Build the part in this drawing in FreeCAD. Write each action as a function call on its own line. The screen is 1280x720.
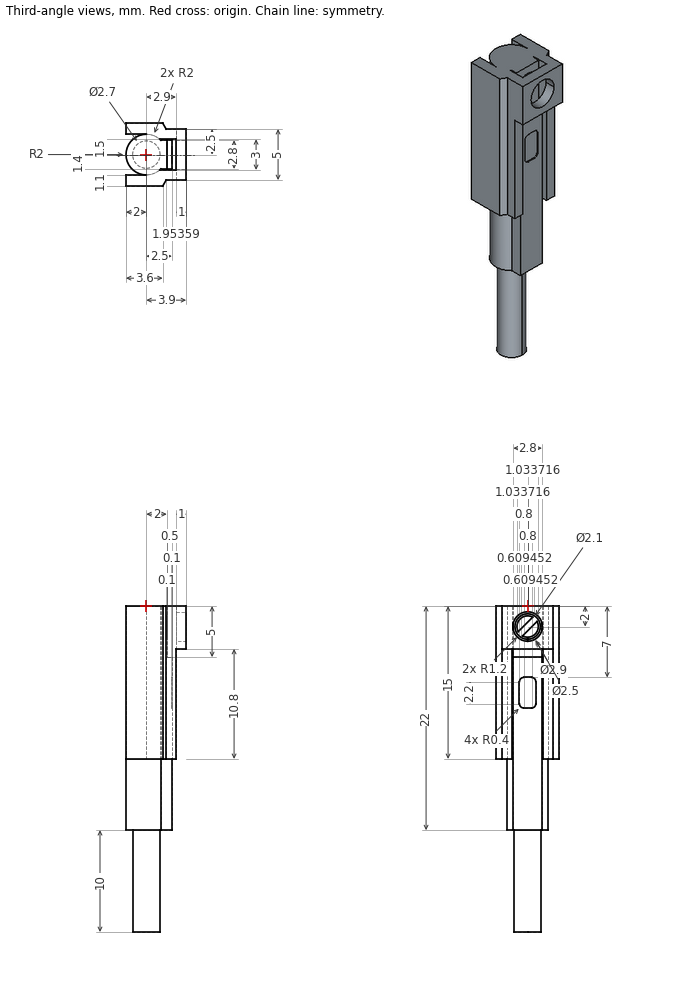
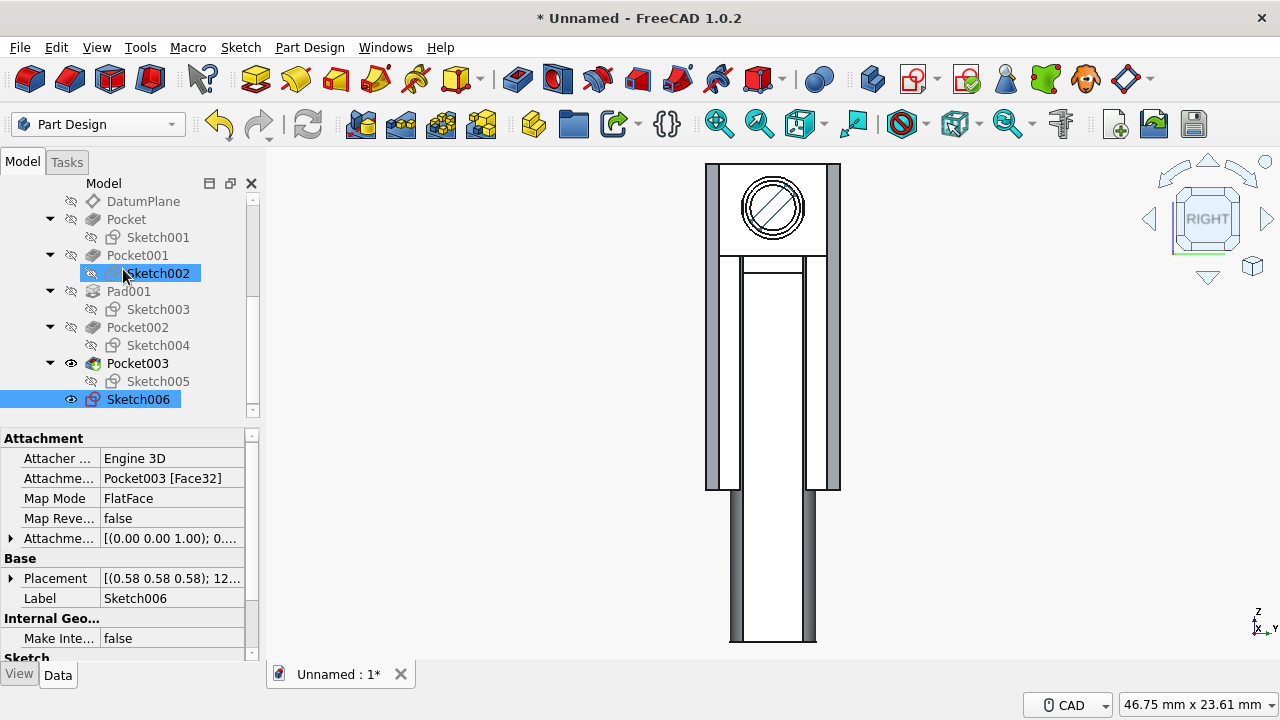
click(518, 80)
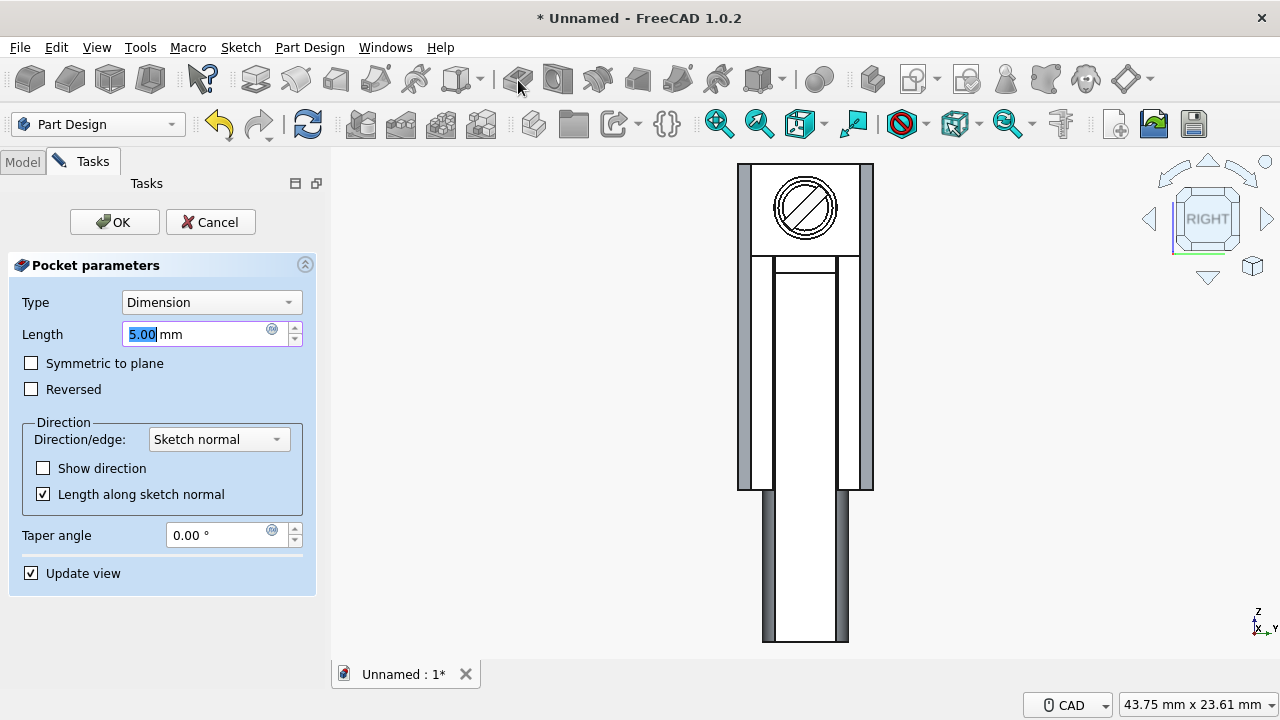
text(0.1)
key(Tab)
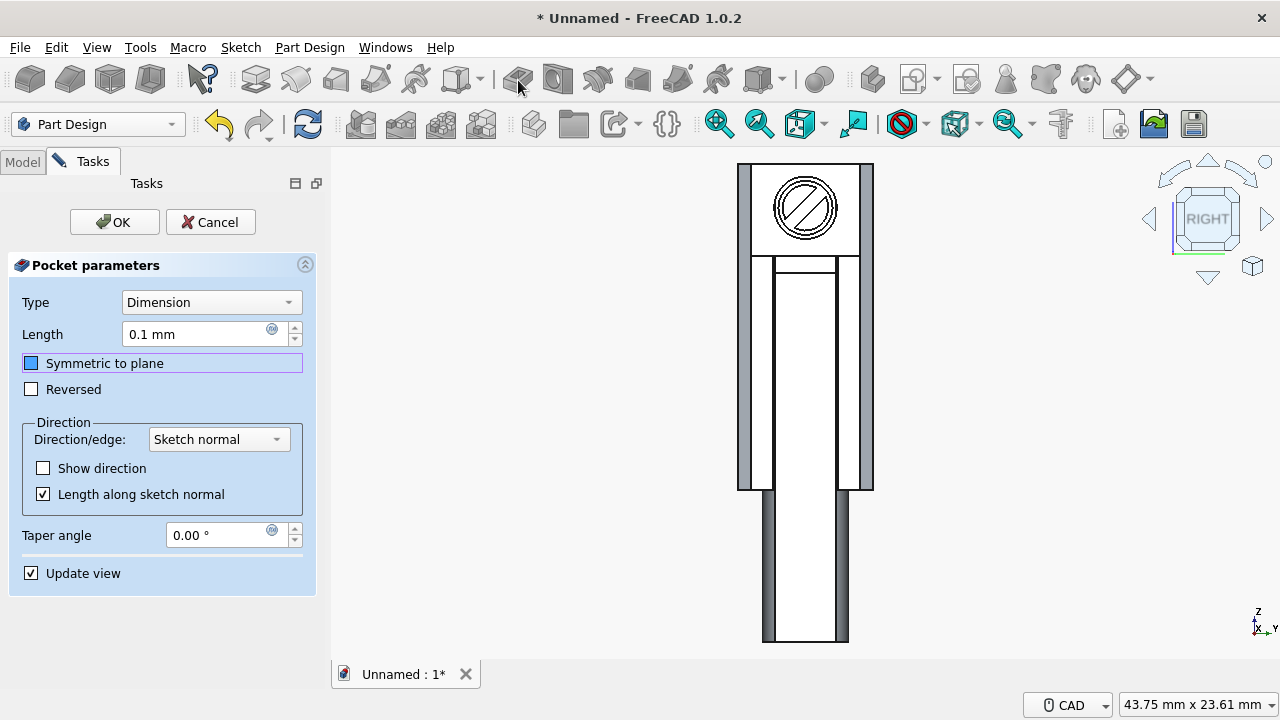
click(115, 222)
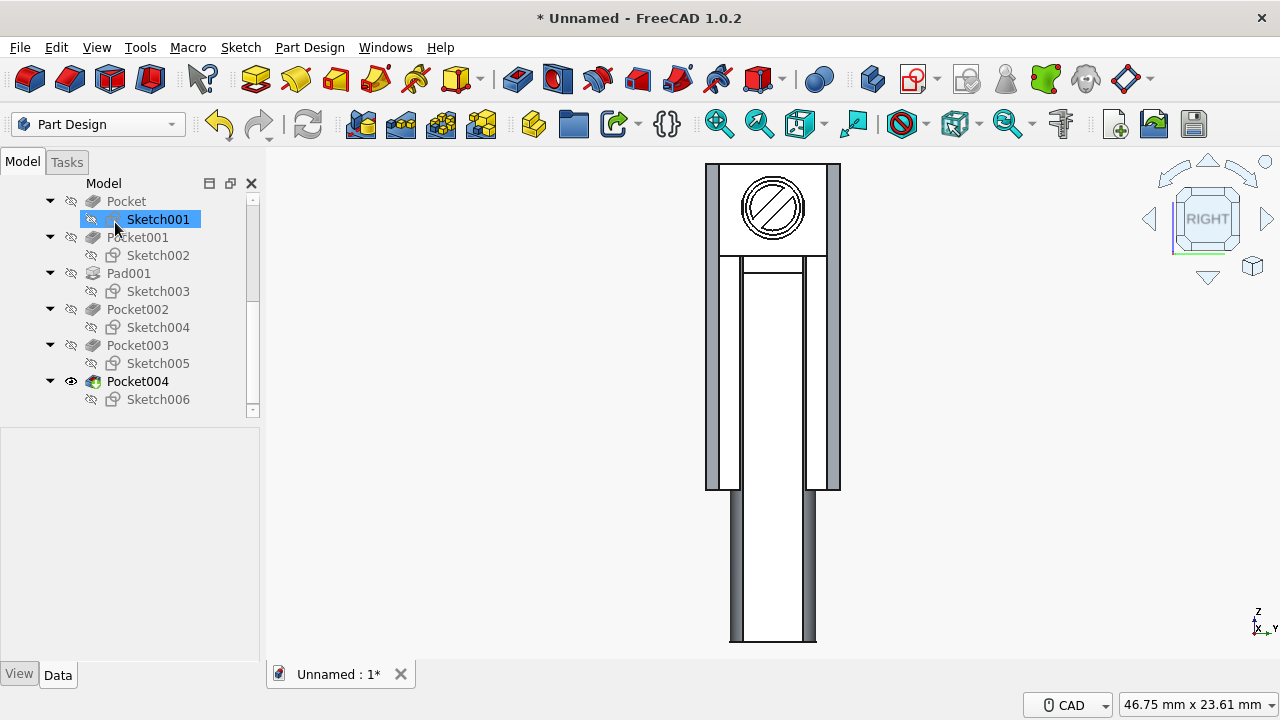
click(773, 351)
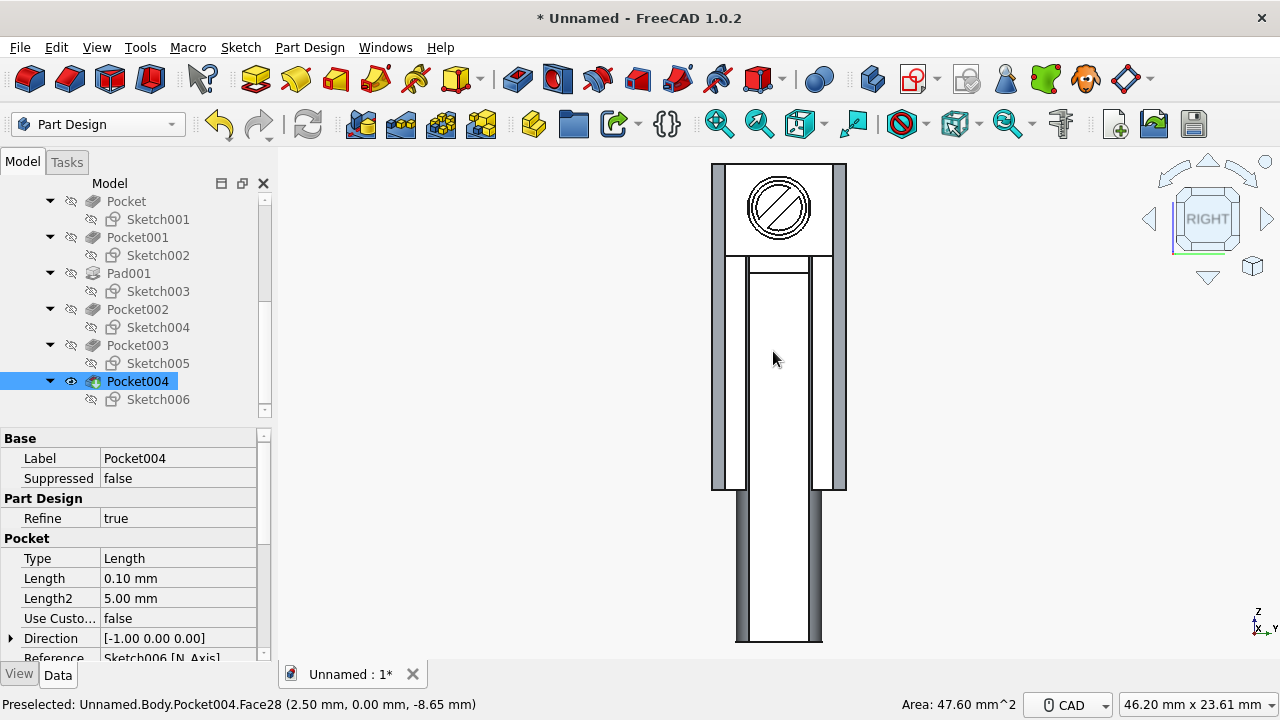
click(914, 80)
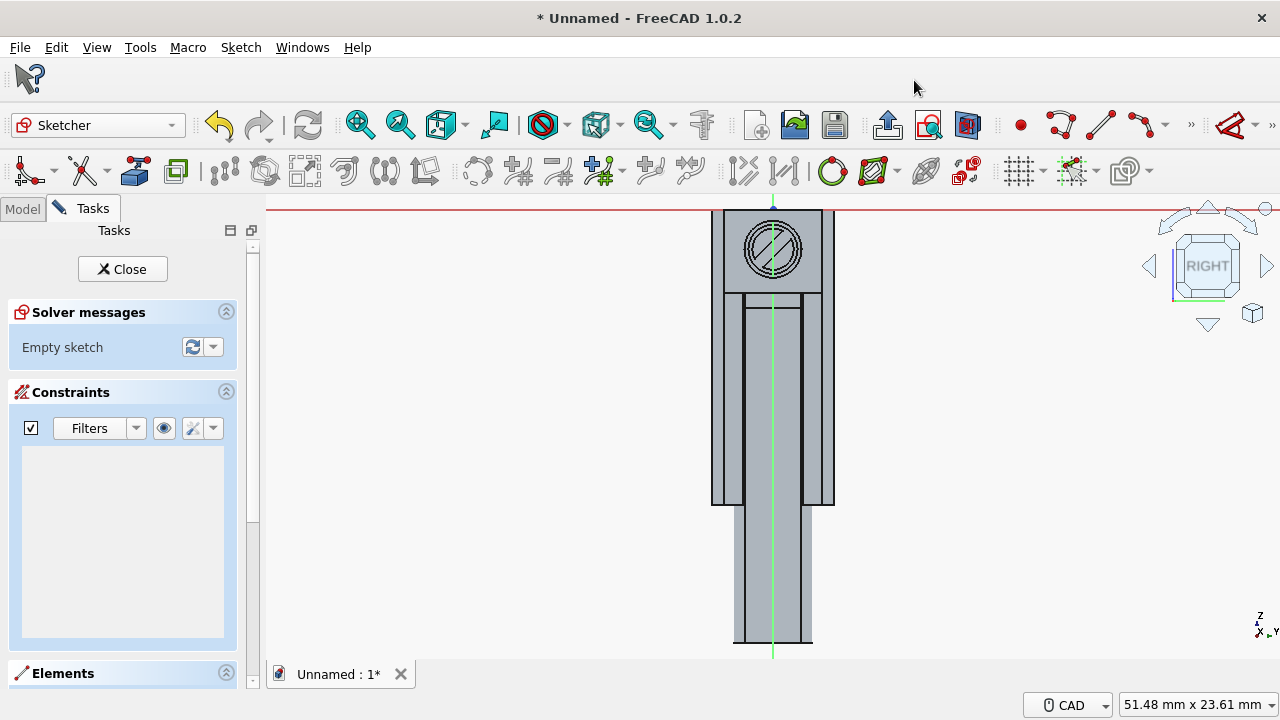
scroll(790, 365, up, 8)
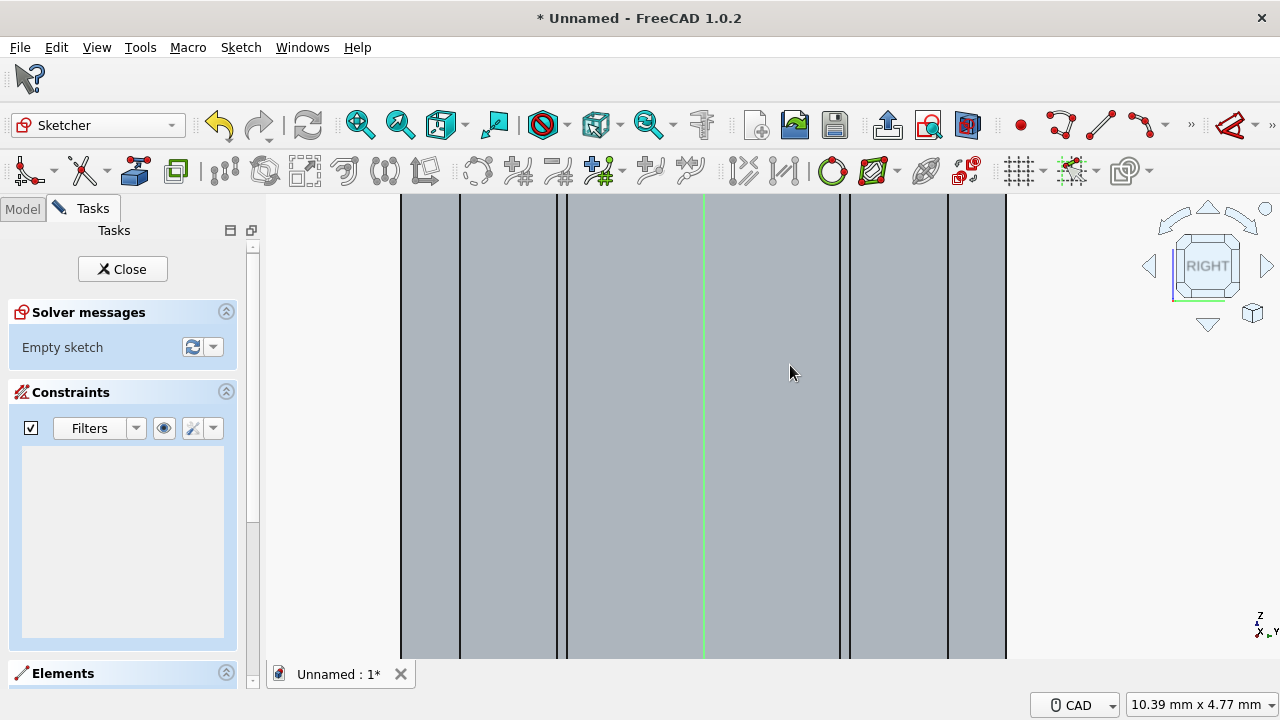
click(1102, 126)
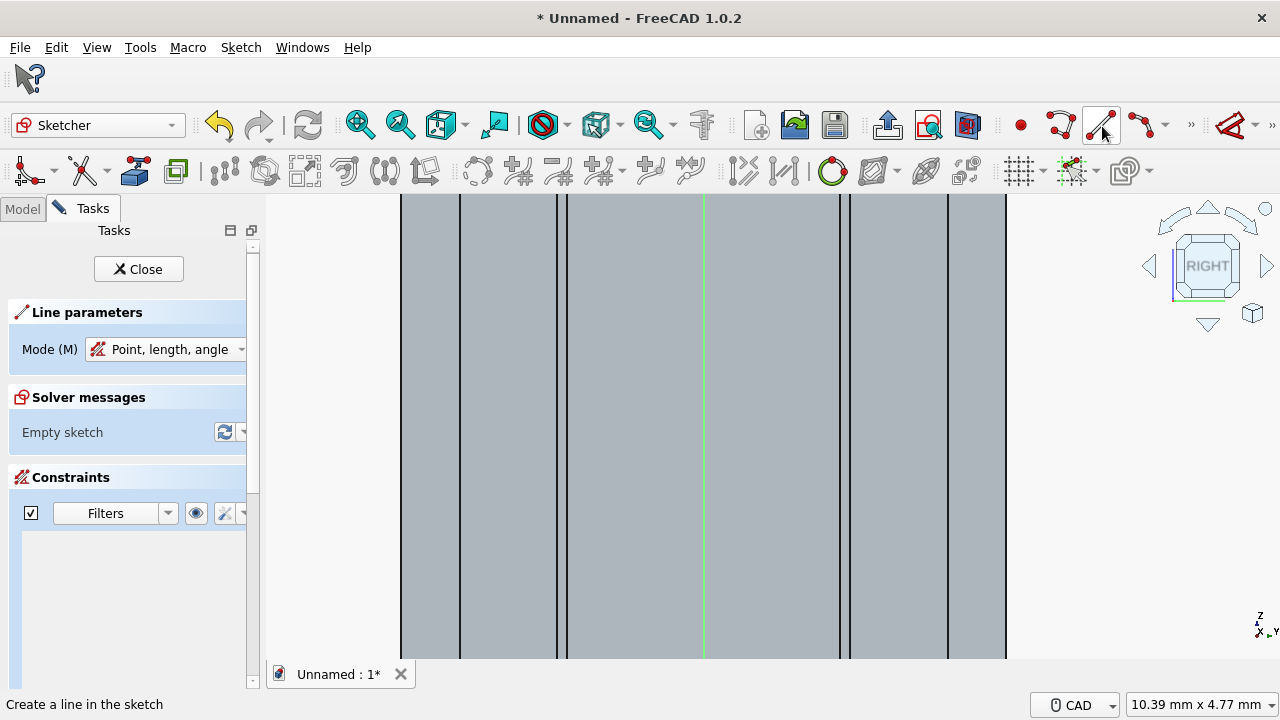
click(626, 317)
click(626, 532)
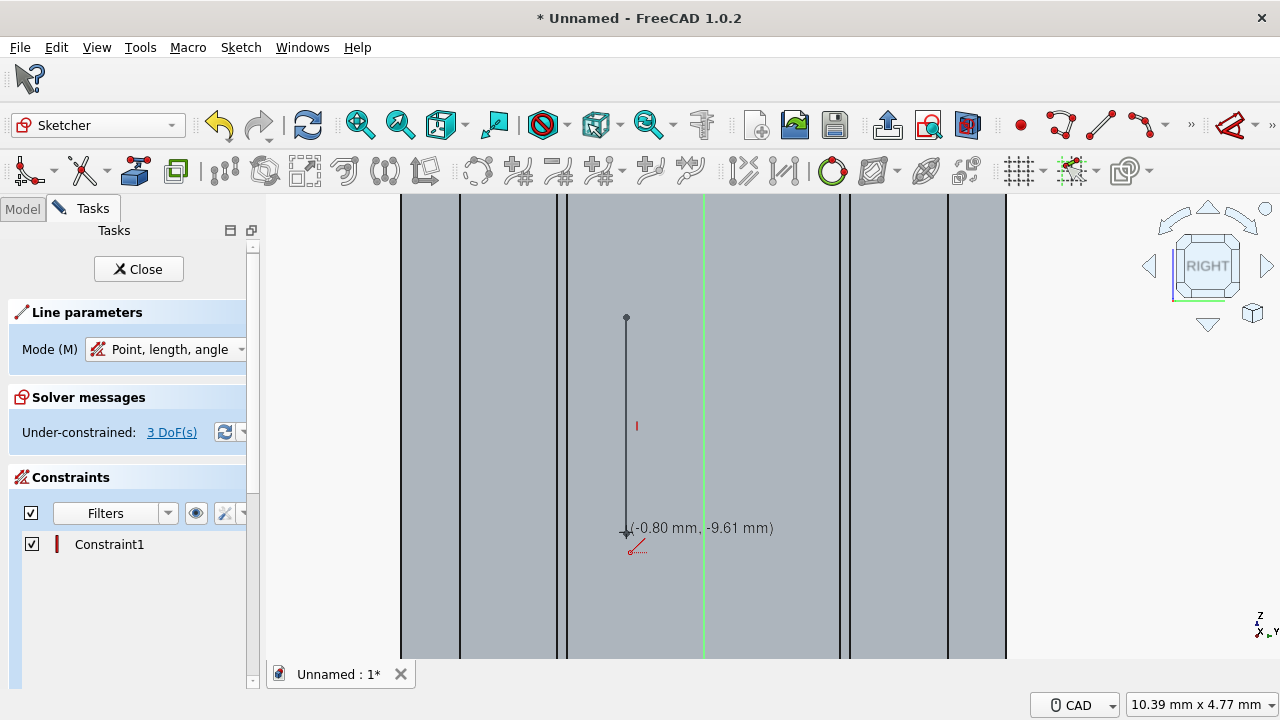
click(665, 571)
click(743, 571)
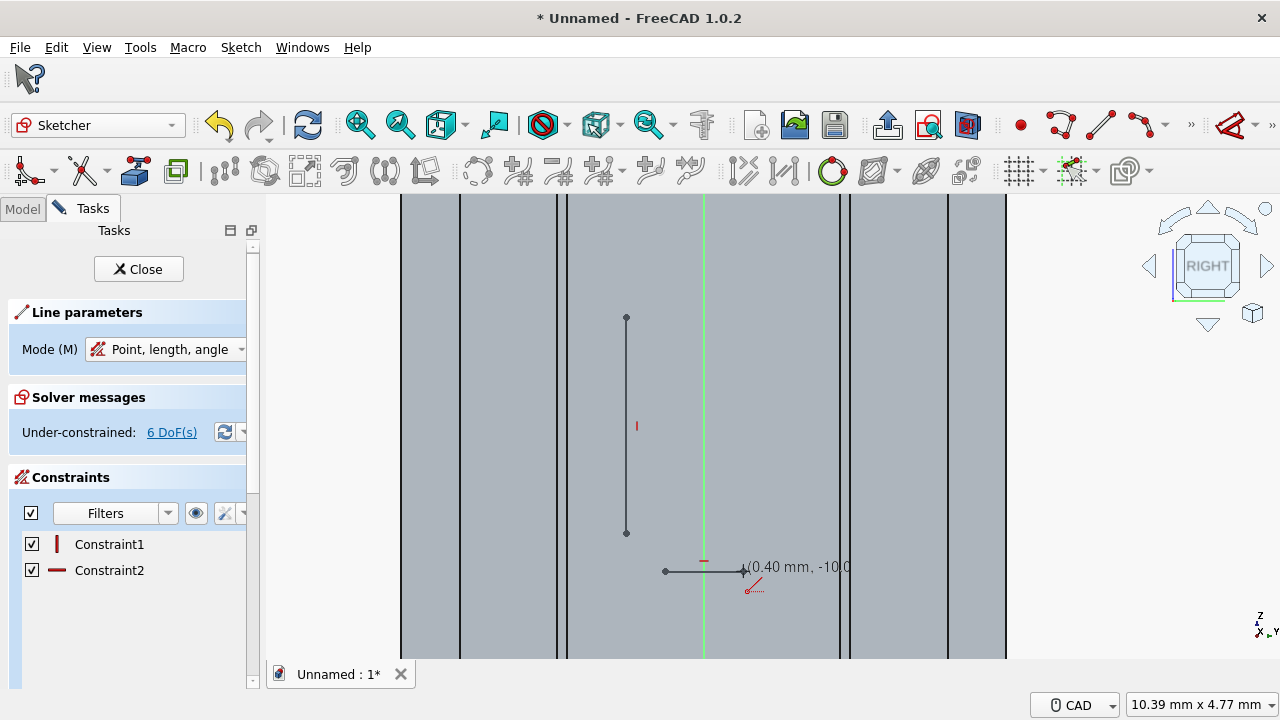
click(782, 532)
click(782, 317)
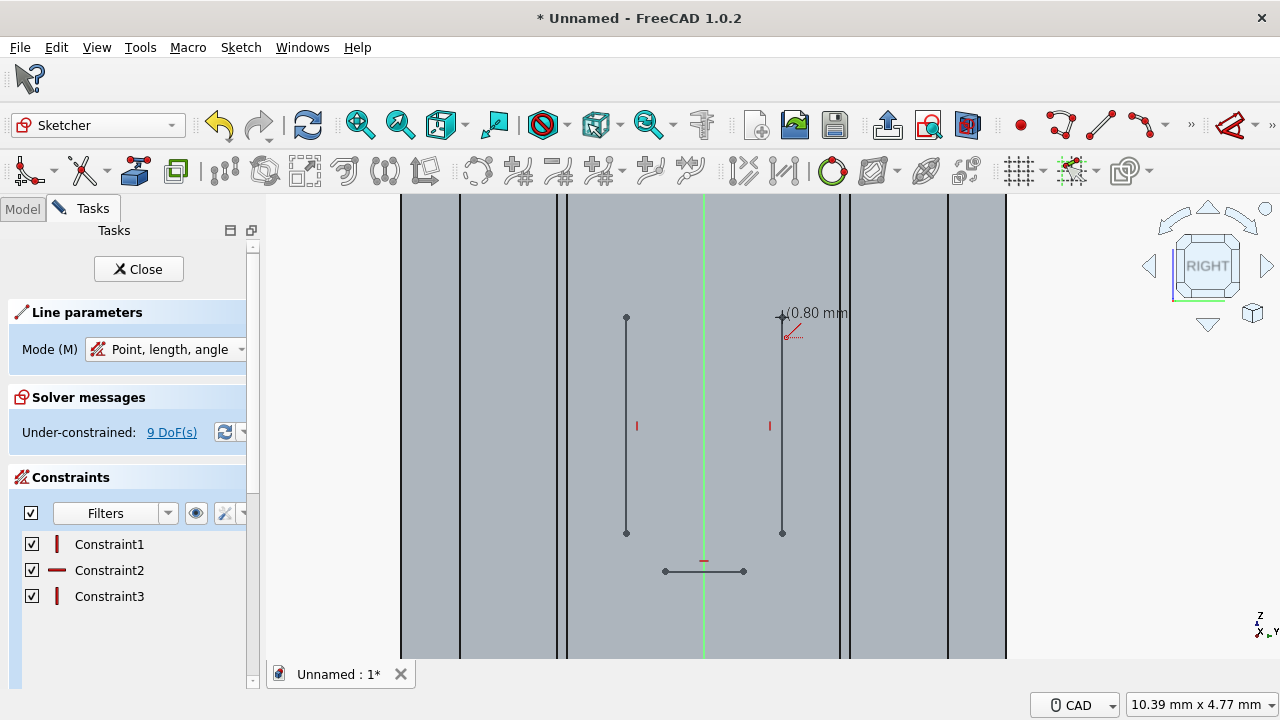
click(743, 278)
click(665, 278)